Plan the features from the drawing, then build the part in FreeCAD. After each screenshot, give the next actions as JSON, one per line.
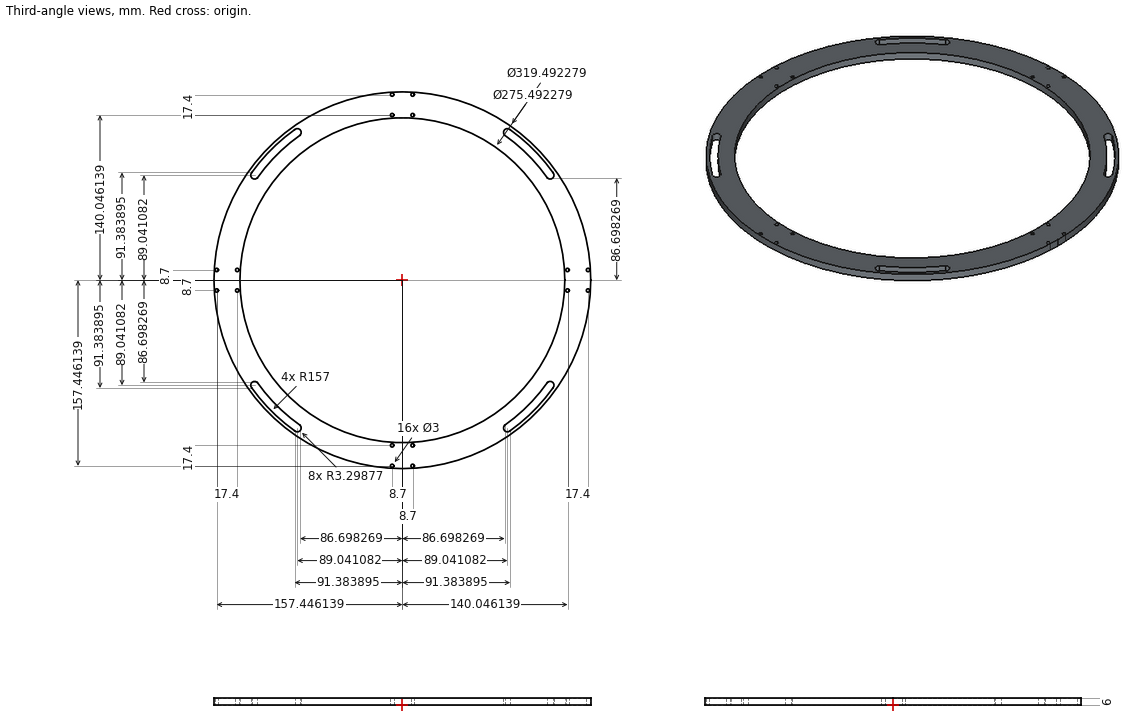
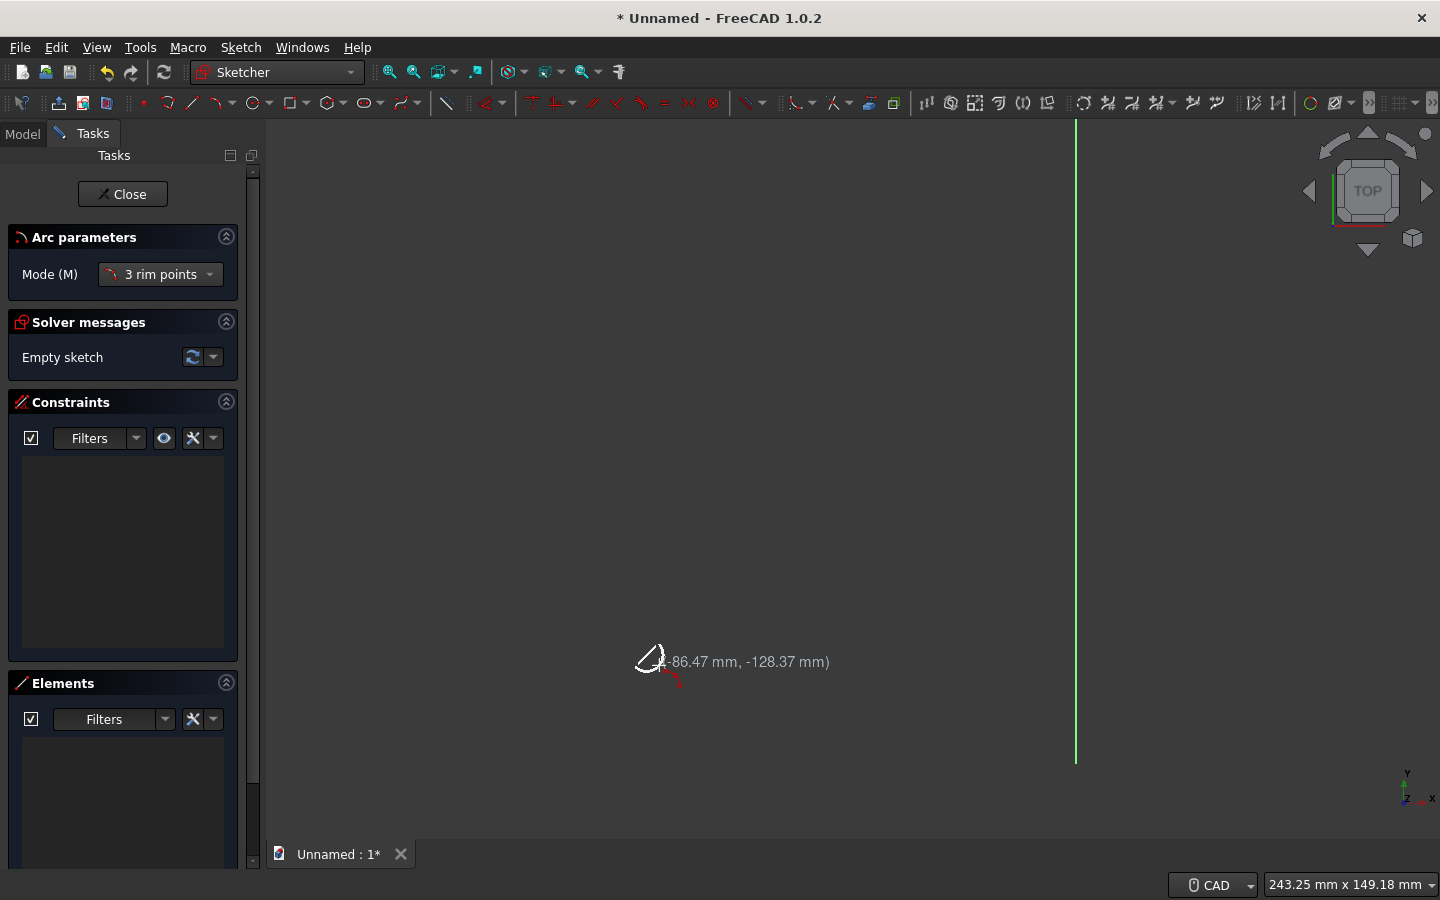
{"action": "left_click", "coordinate": [657, 663]}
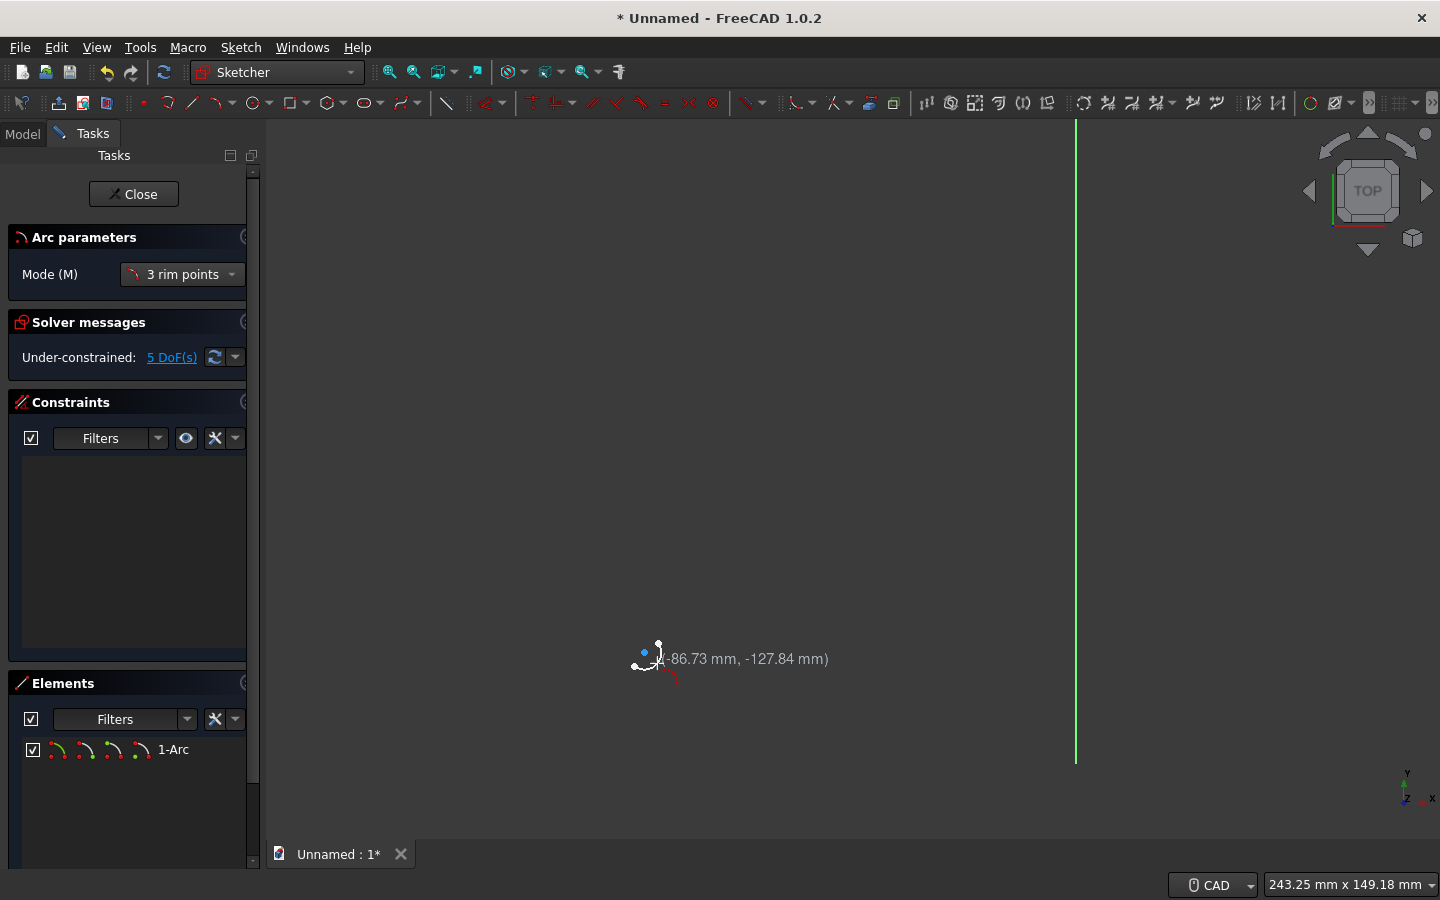
{"action": "left_click", "coordinate": [635, 667]}
{"action": "left_click", "coordinate": [459, 488]}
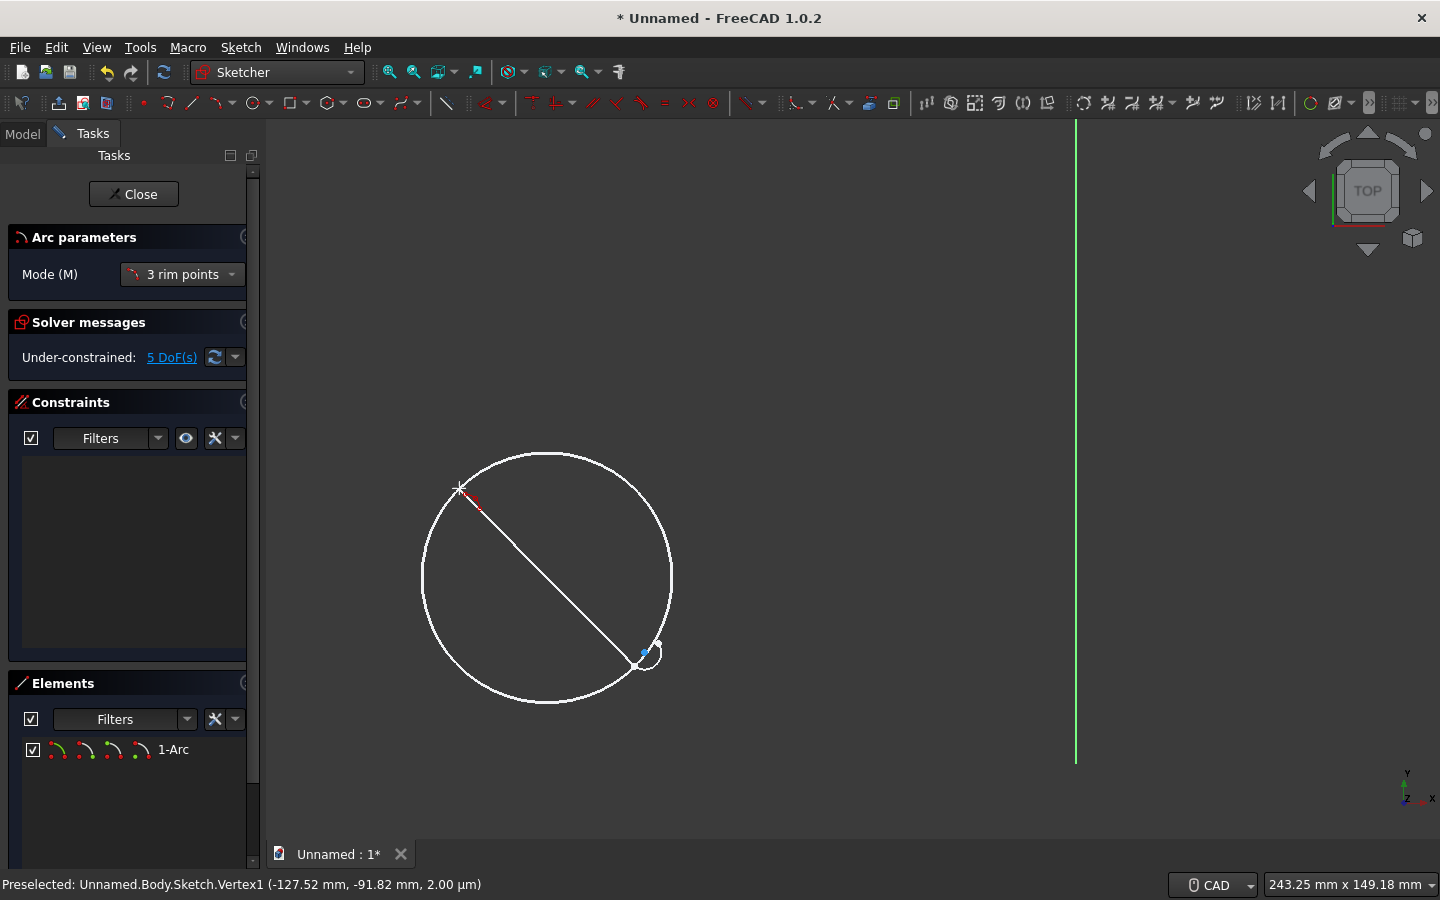
{"action": "scroll", "coordinate": [540, 583], "scroll_direction": "up", "scroll_amount": 3}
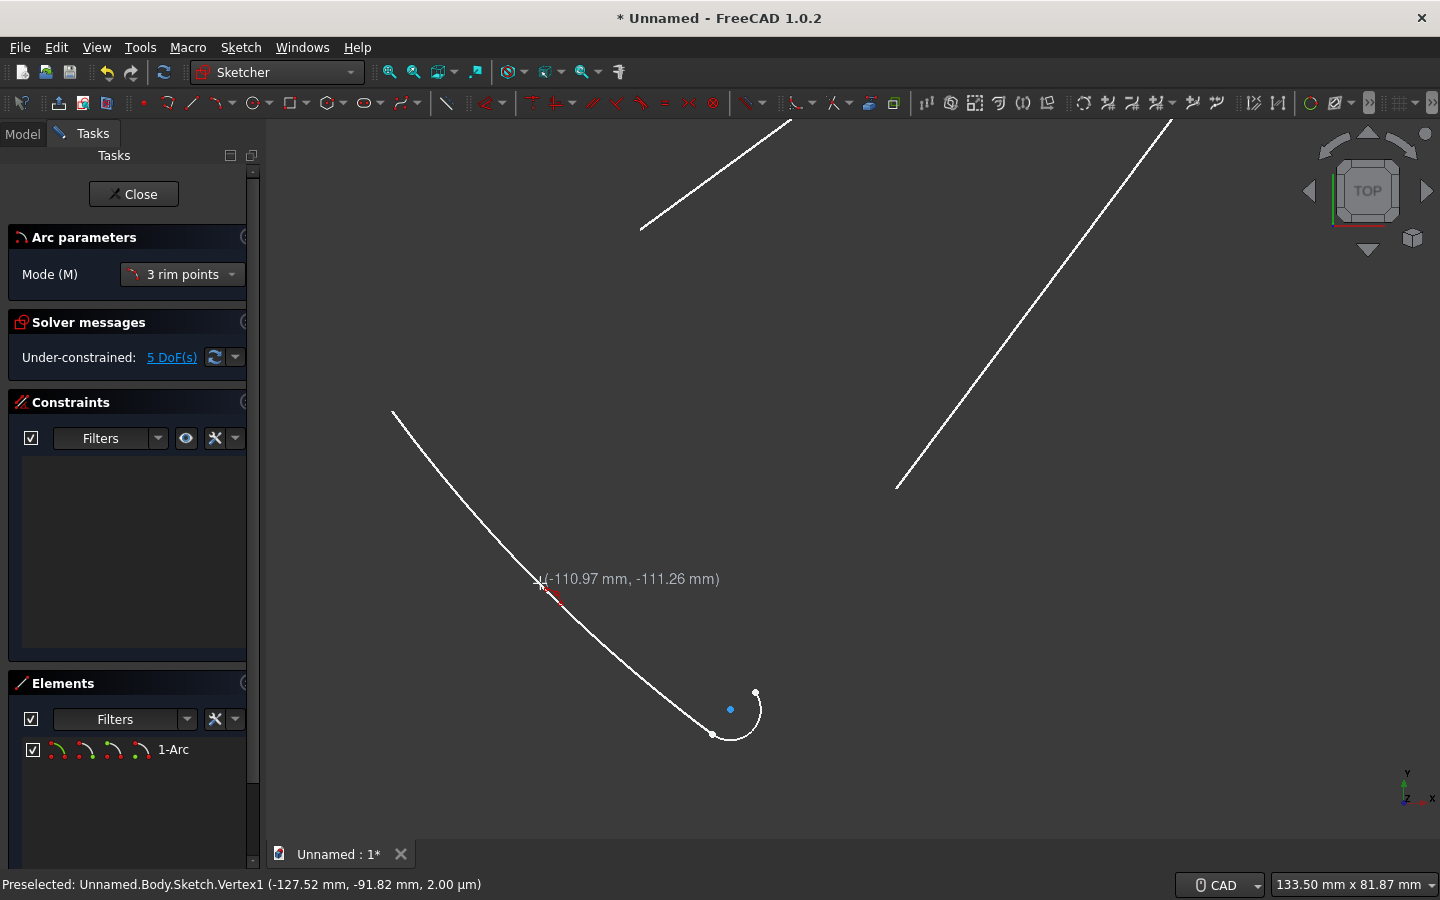
{"action": "left_click", "coordinate": [539, 582]}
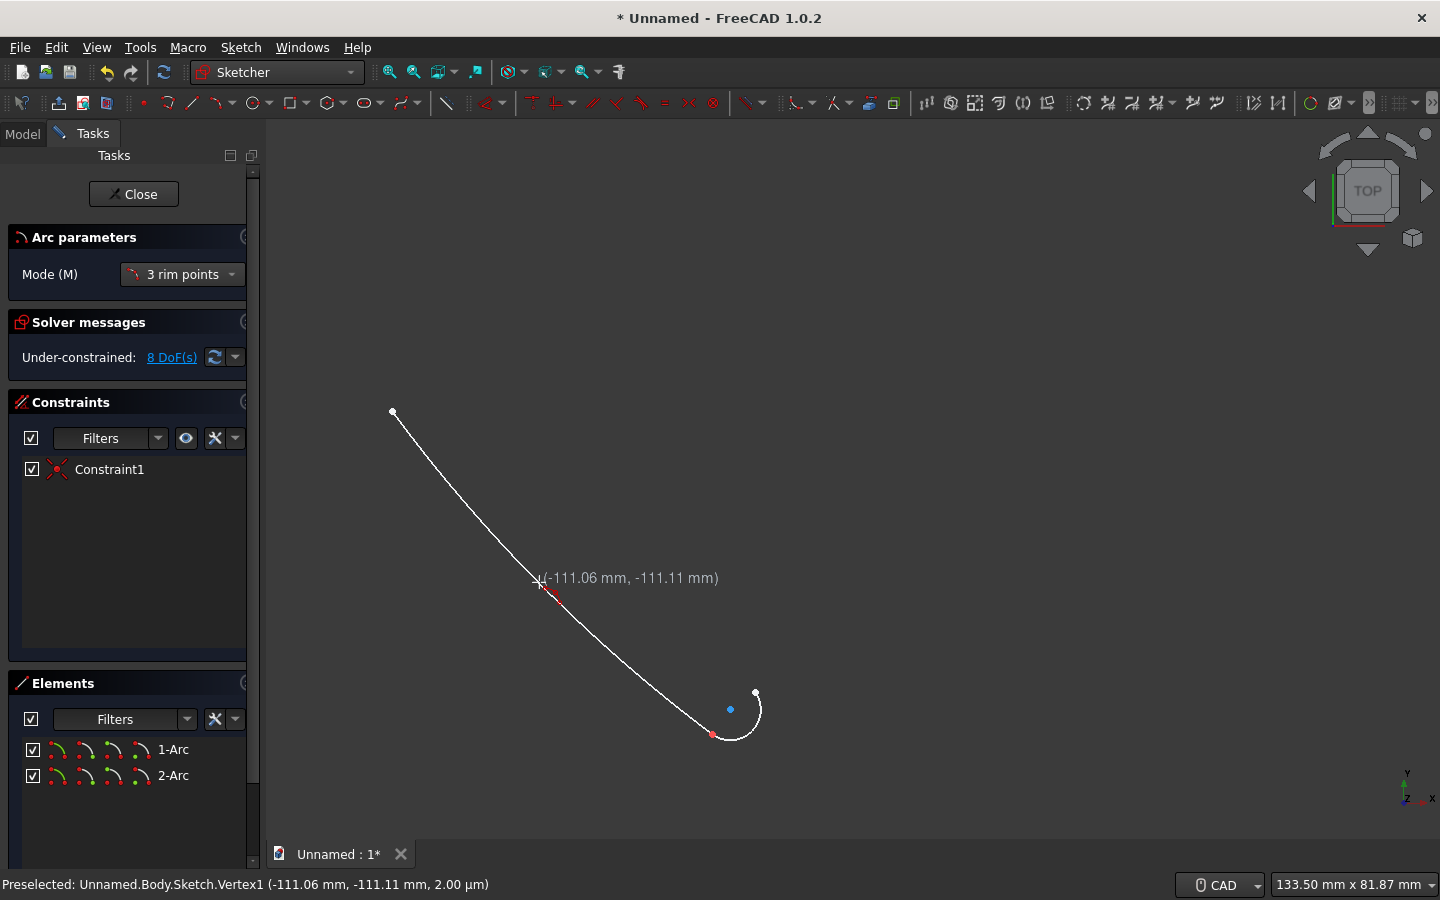
{"action": "scroll", "coordinate": [640, 652], "scroll_direction": "down", "scroll_amount": 9}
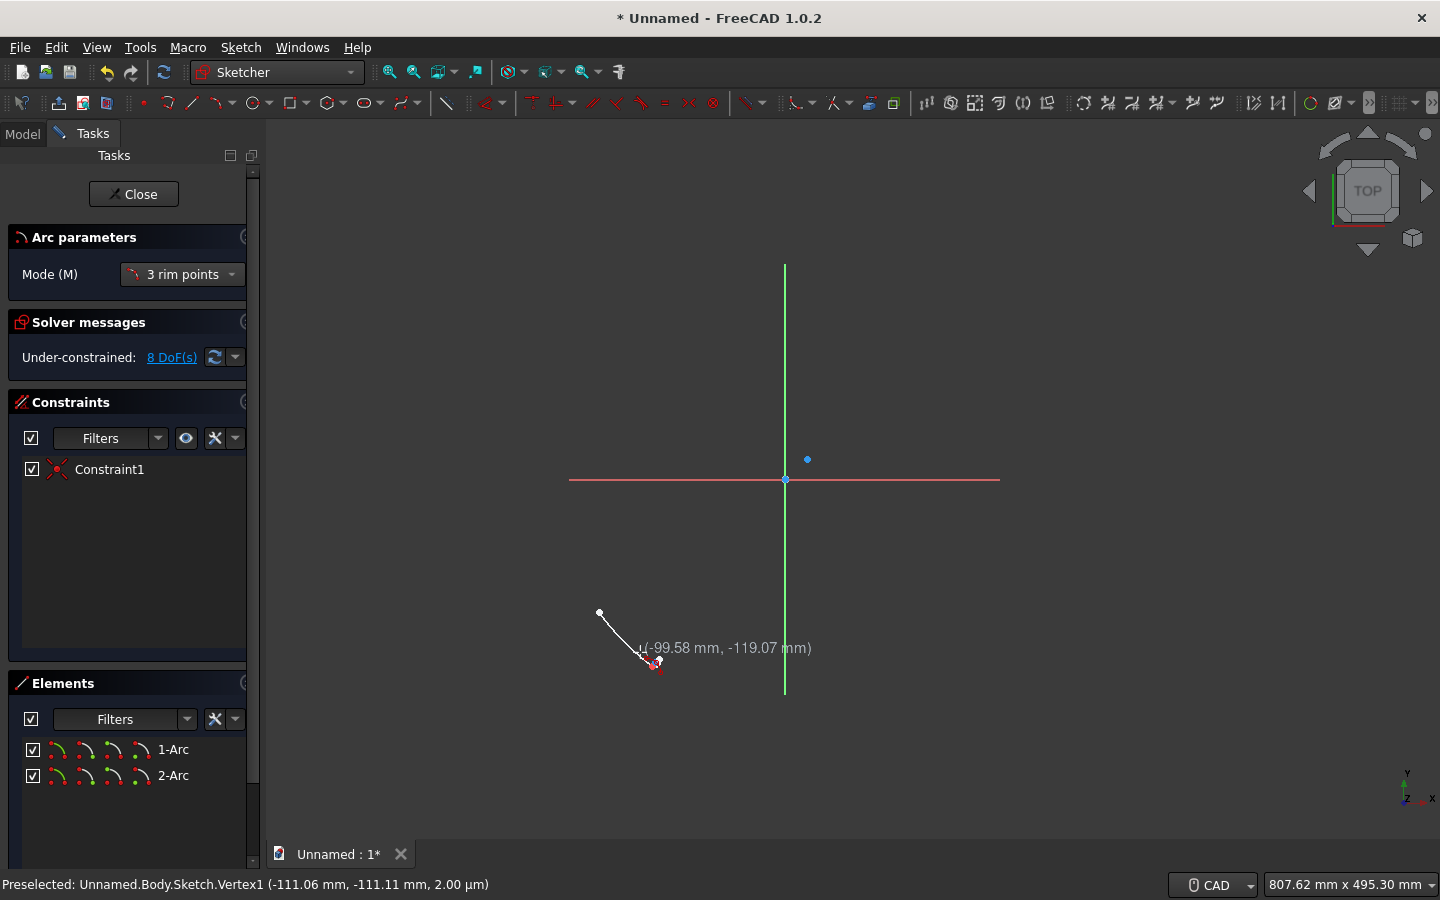
{"action": "left_click", "coordinate": [599, 613]}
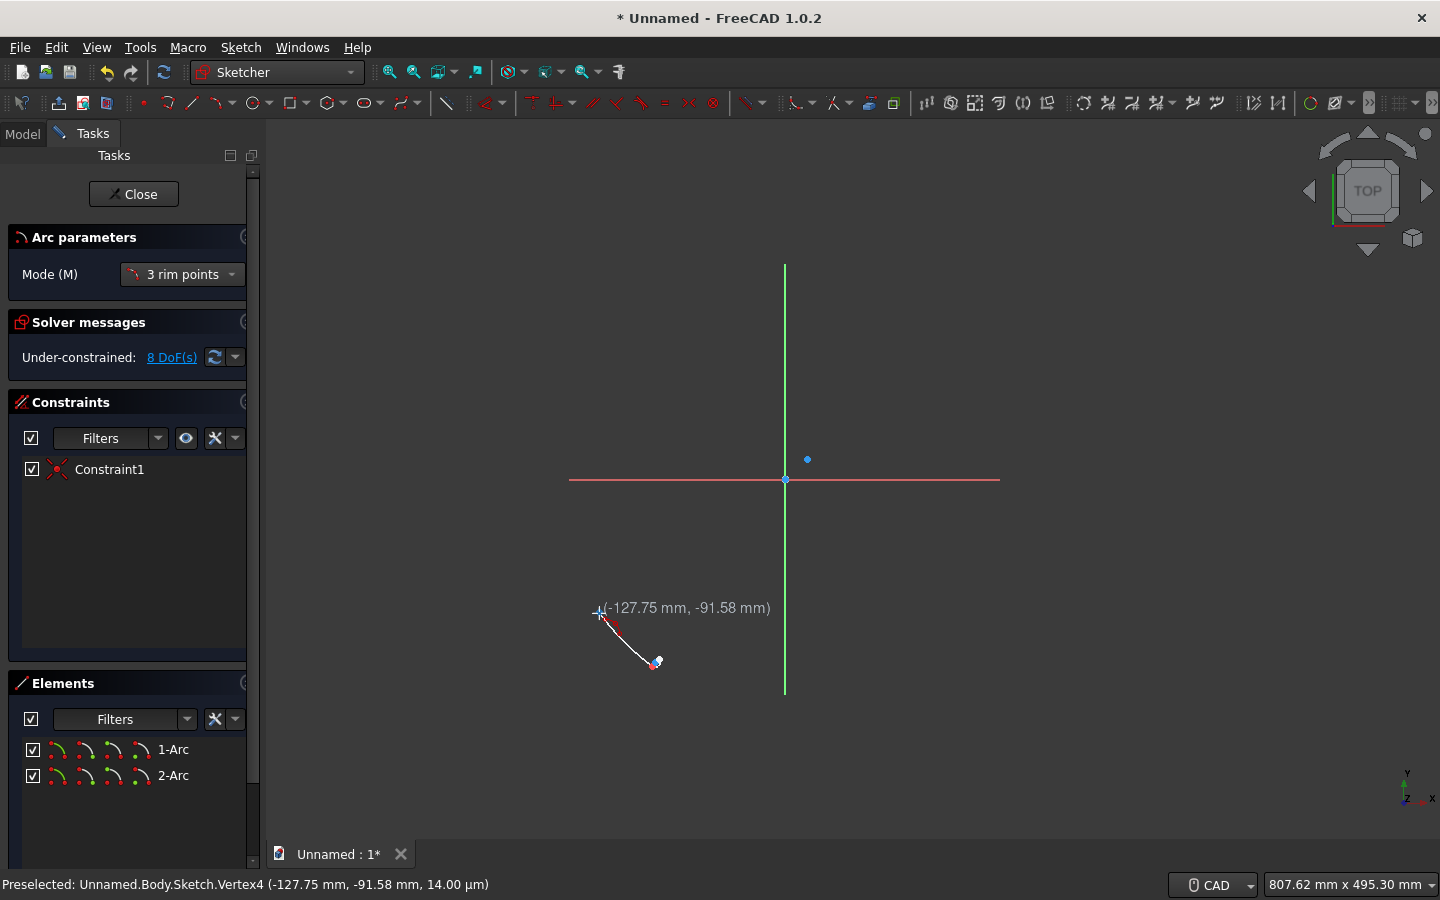
{"action": "scroll", "coordinate": [606, 606], "scroll_direction": "up", "scroll_amount": 3}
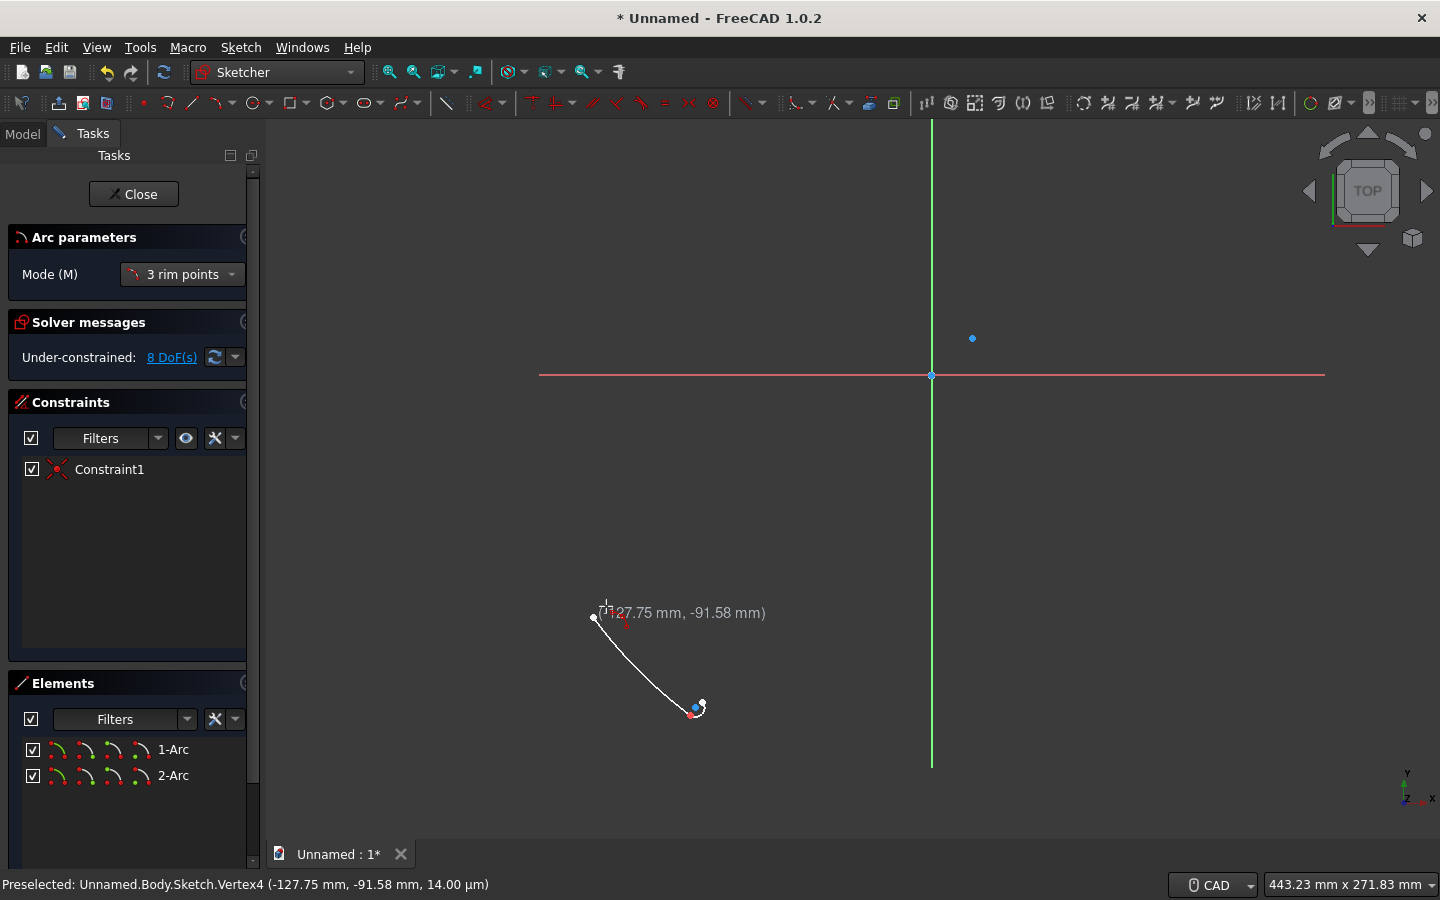
{"action": "left_click", "coordinate": [606, 605]}